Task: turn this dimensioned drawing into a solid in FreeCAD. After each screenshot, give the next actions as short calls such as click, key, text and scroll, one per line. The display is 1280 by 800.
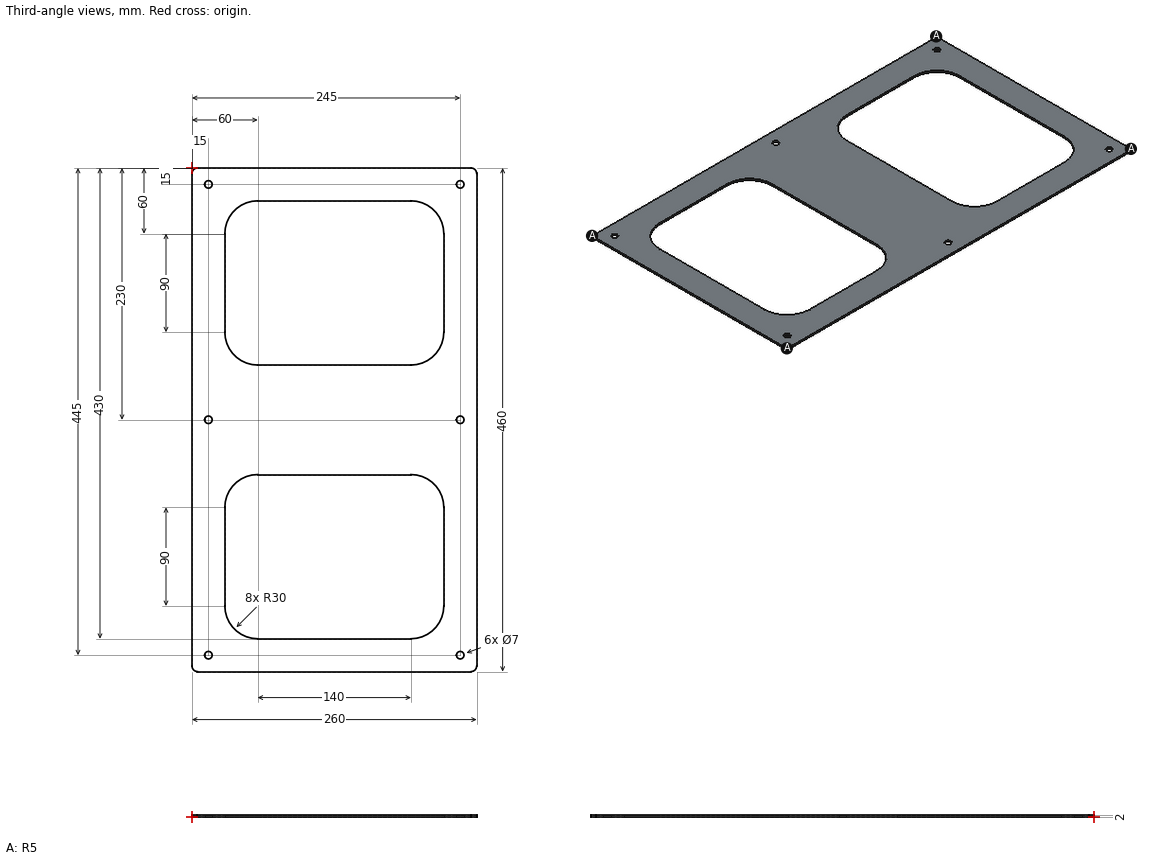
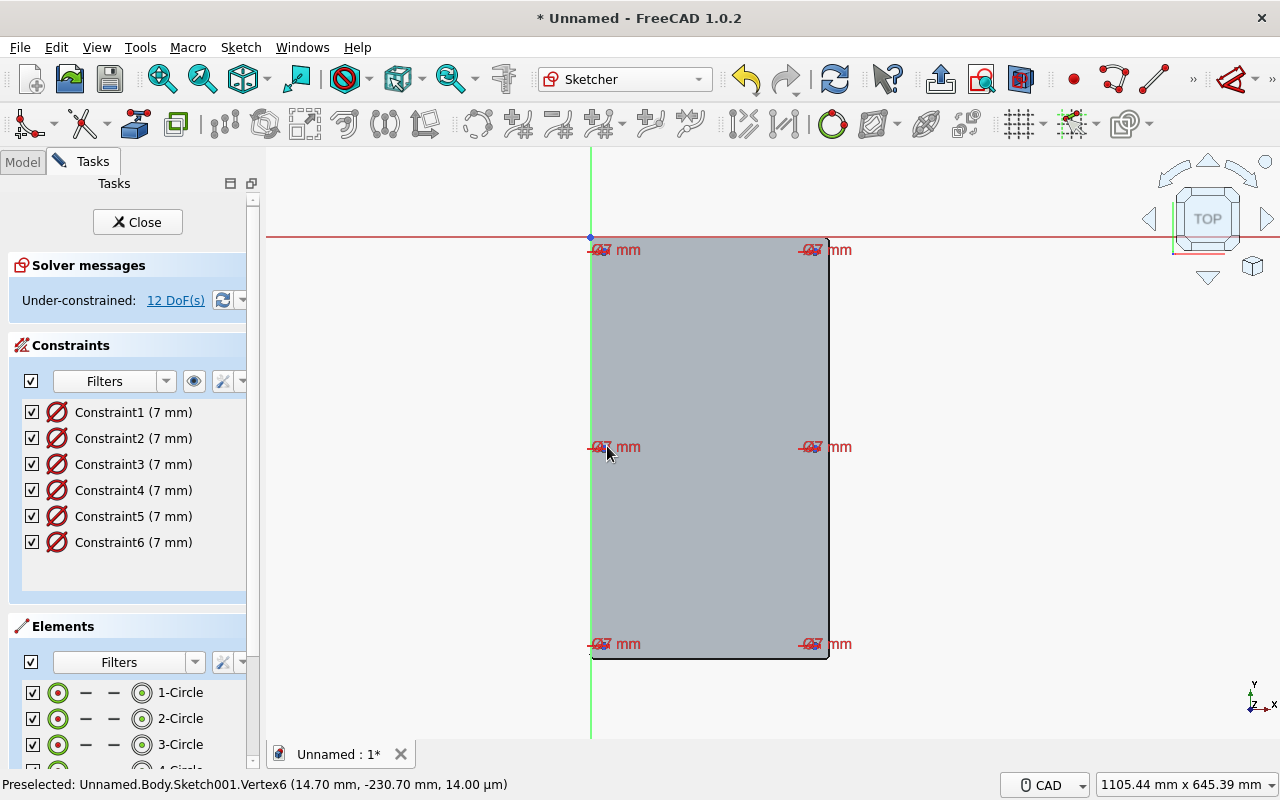
click(815, 646)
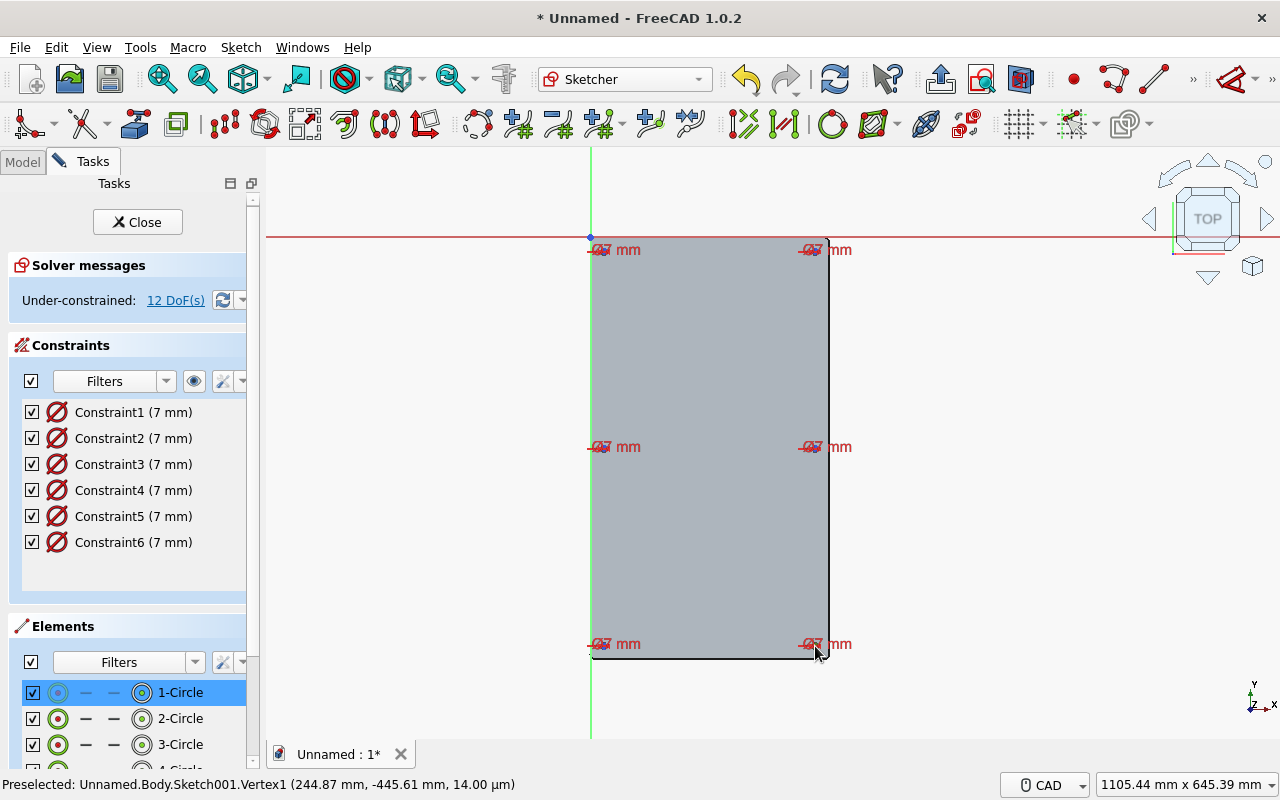
click(604, 646)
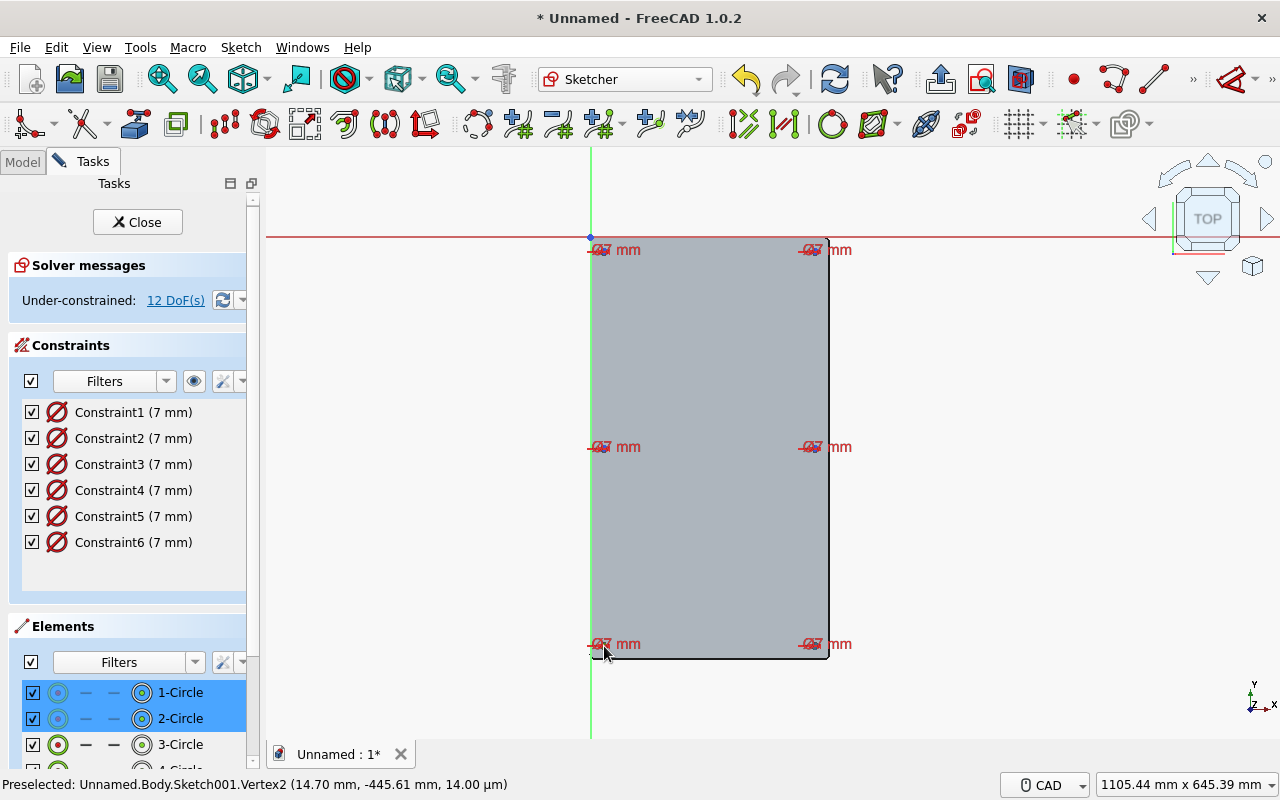
key(h)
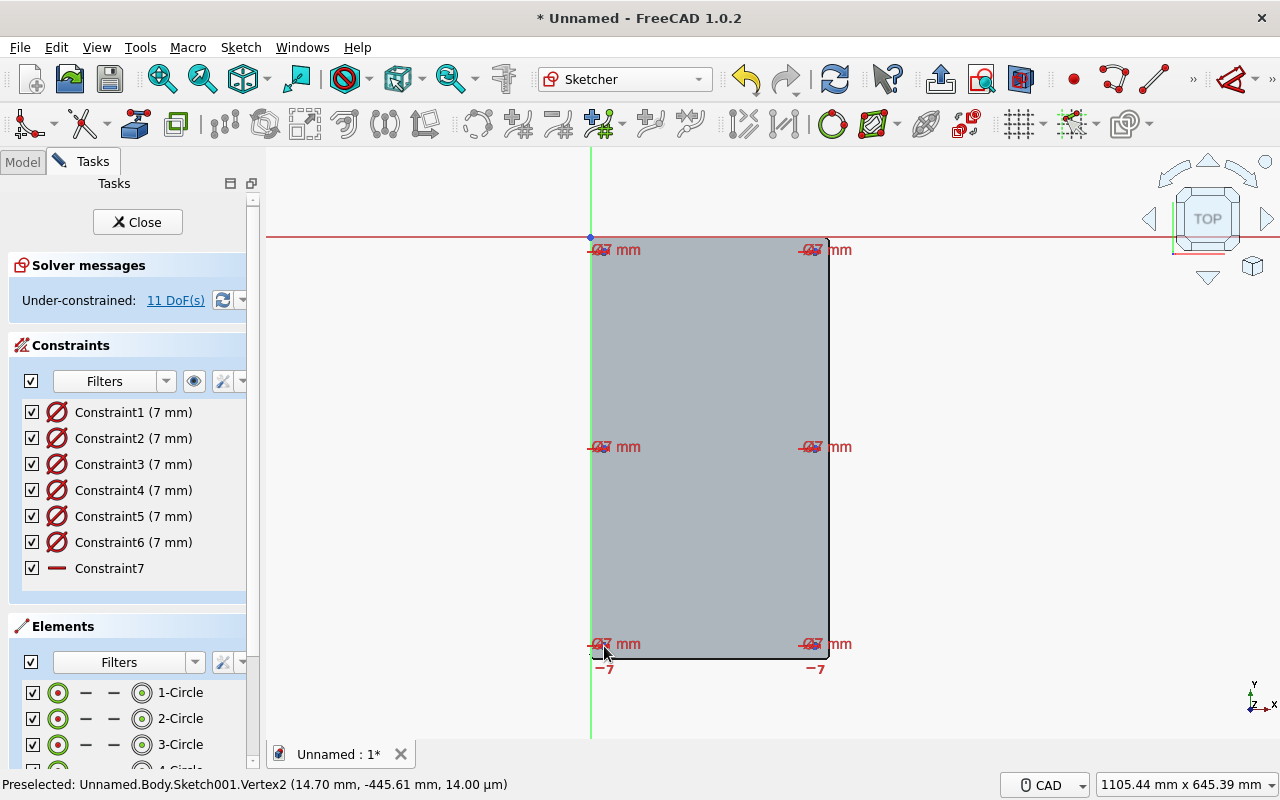
click(815, 646)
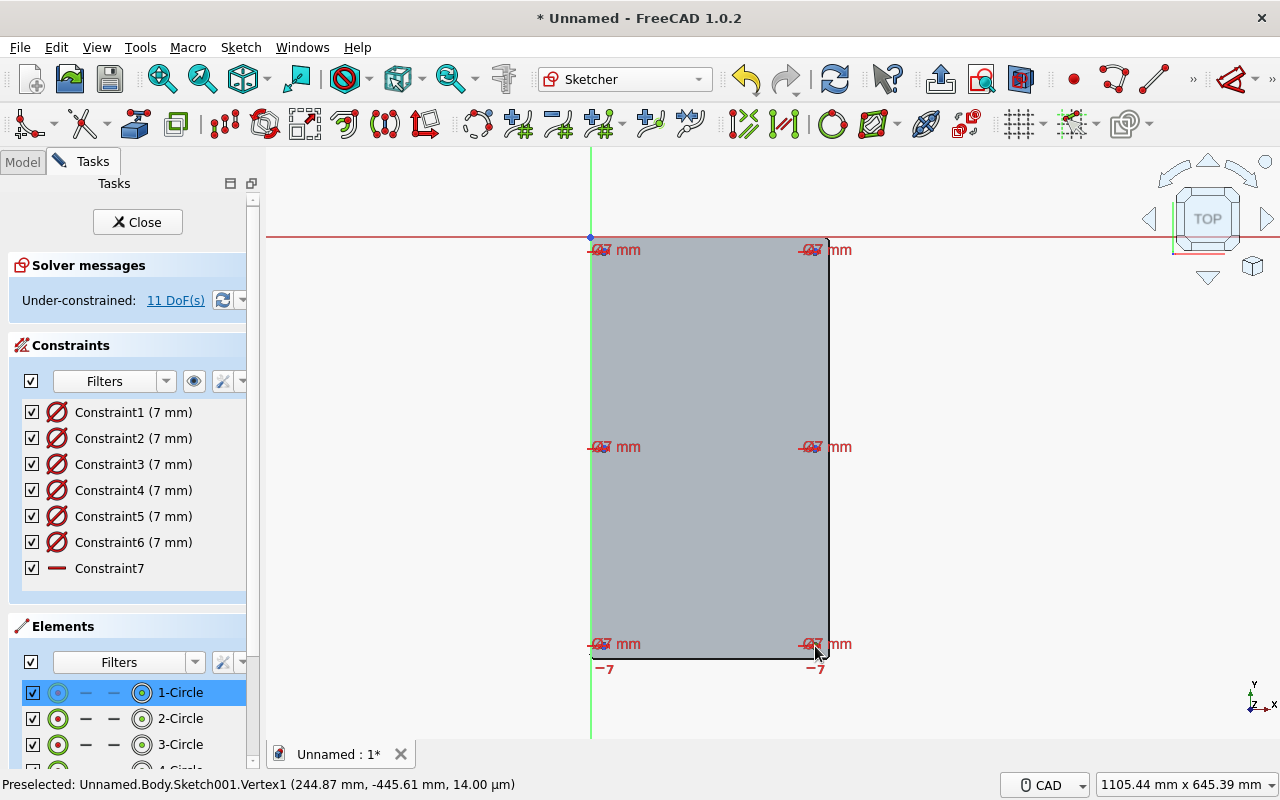
click(815, 252)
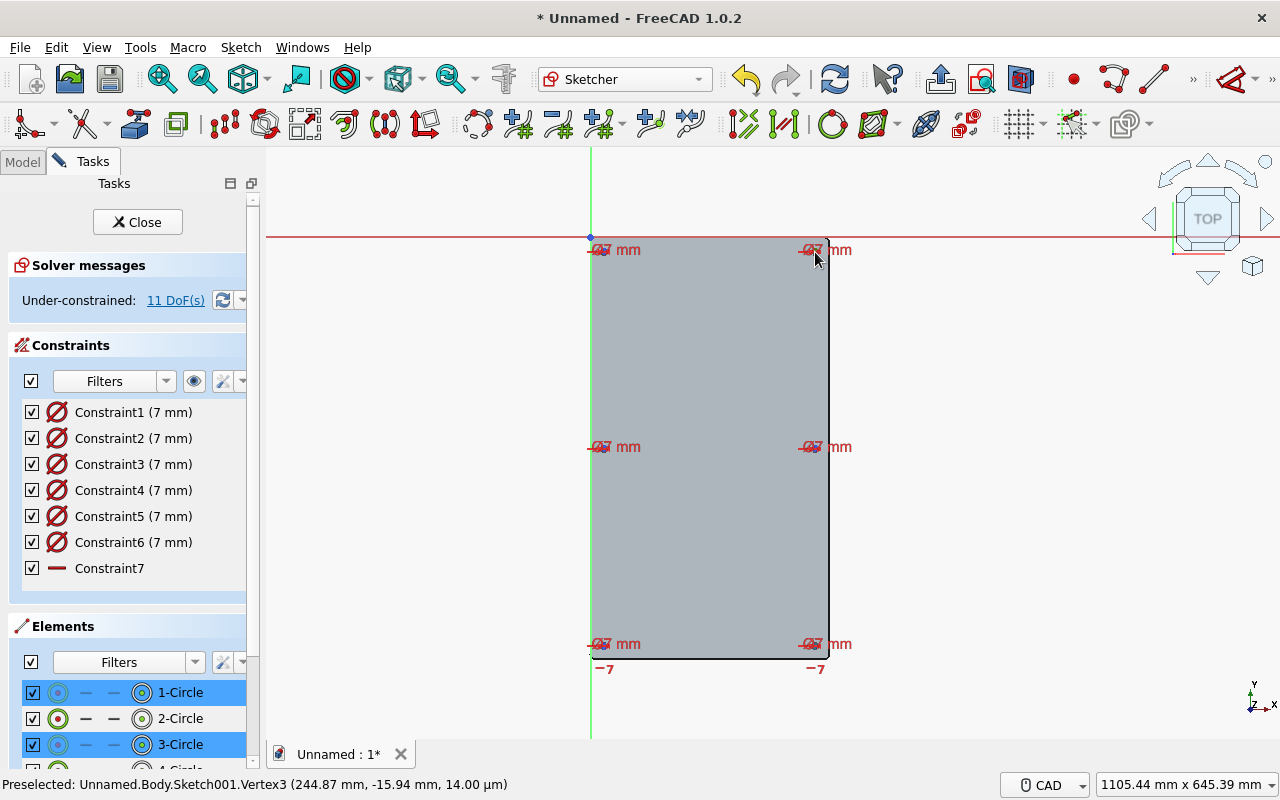
key(v)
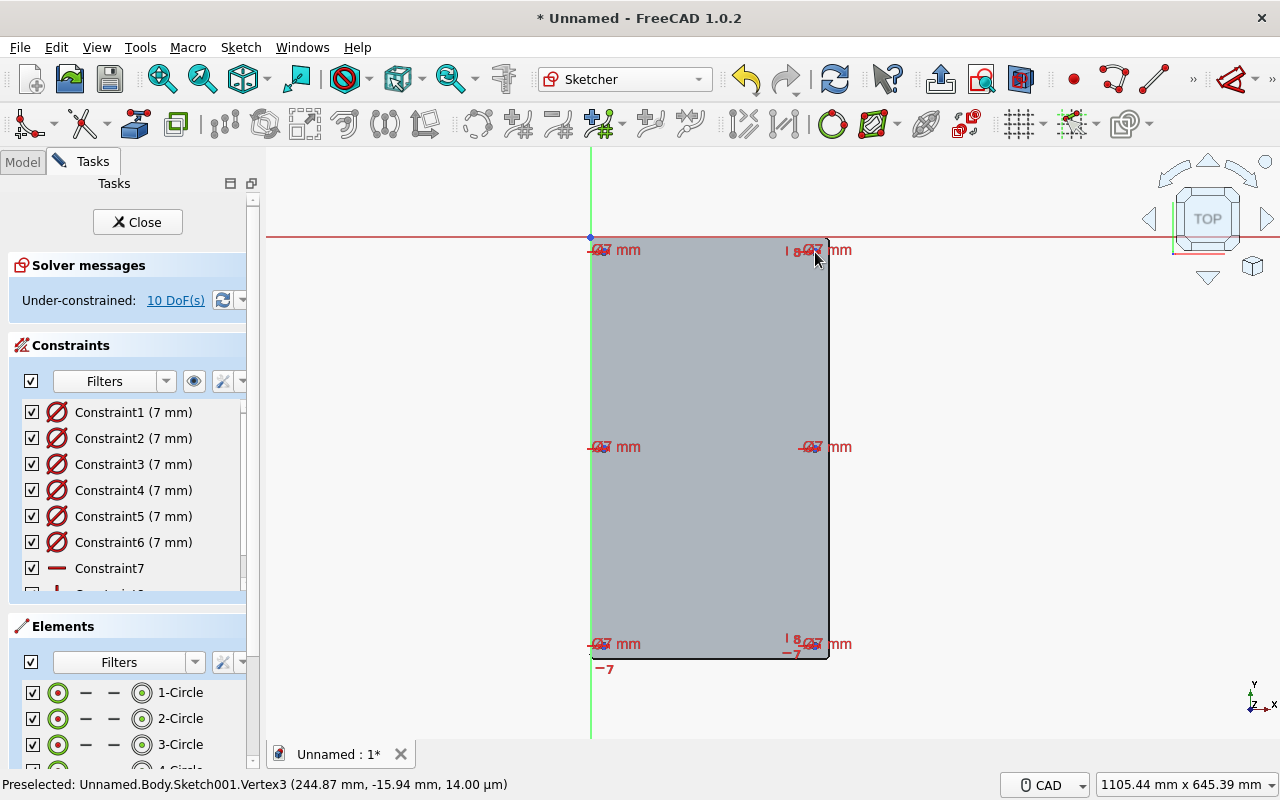
click(604, 646)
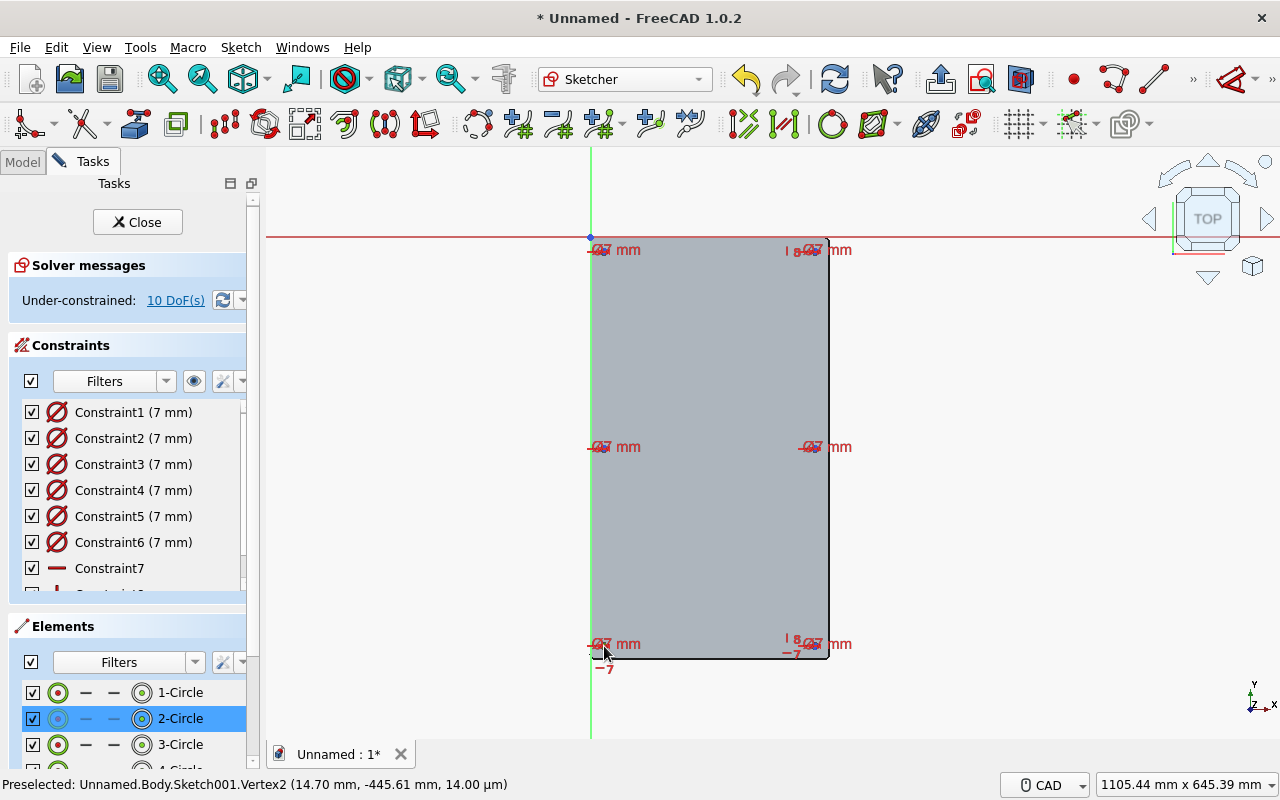
click(604, 252)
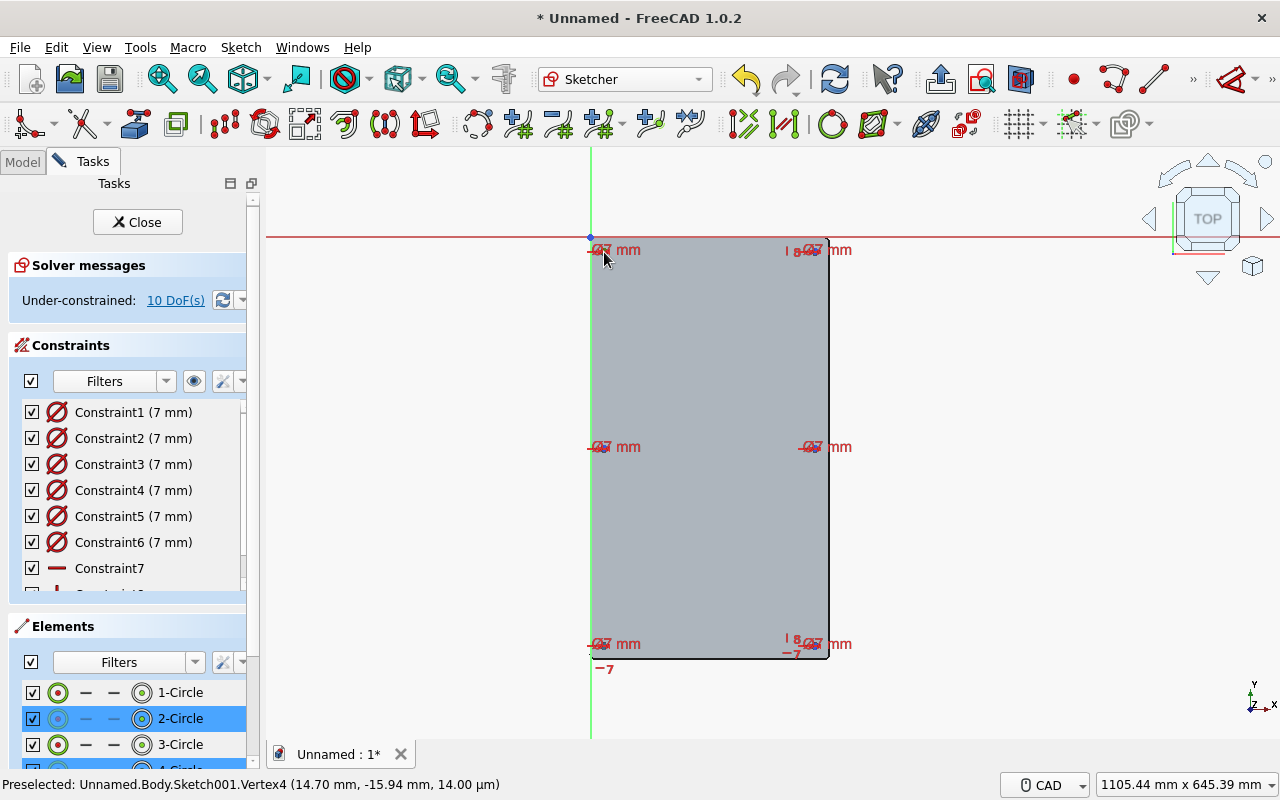
key(v)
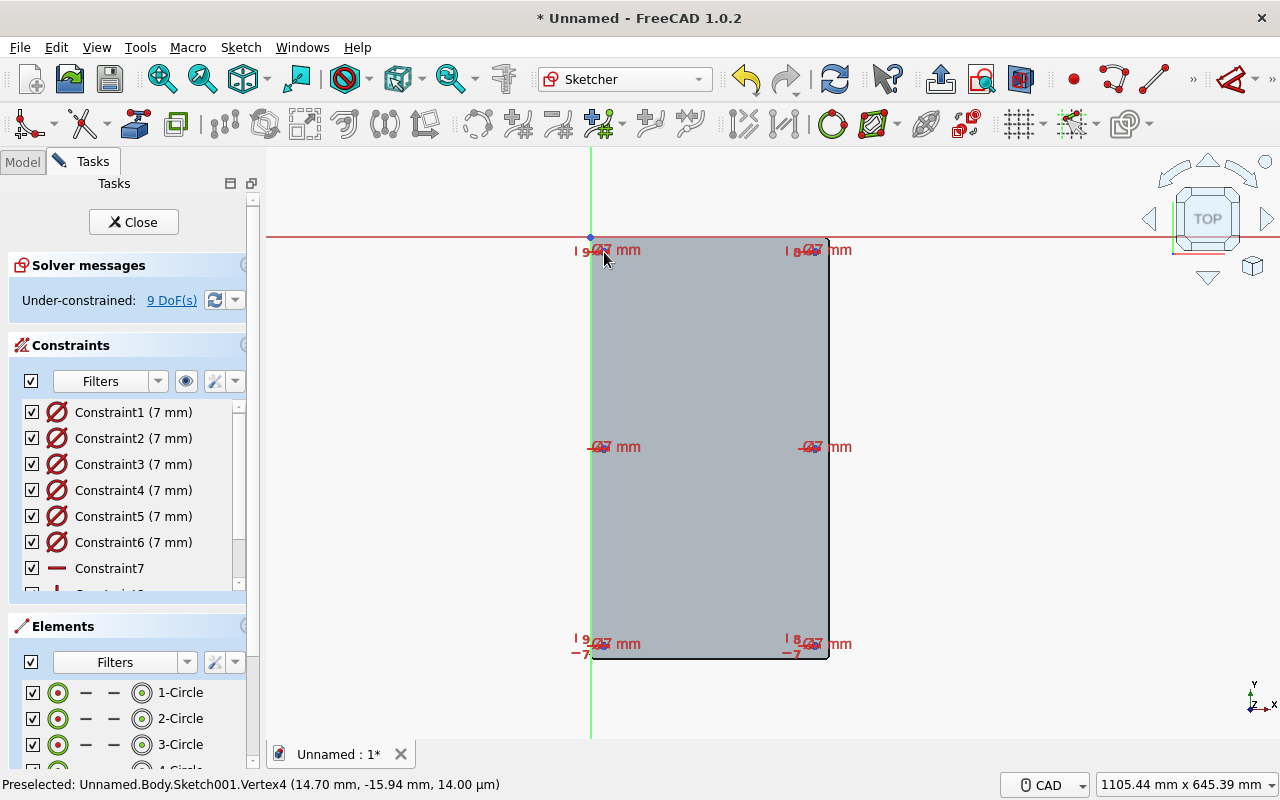
click(815, 252)